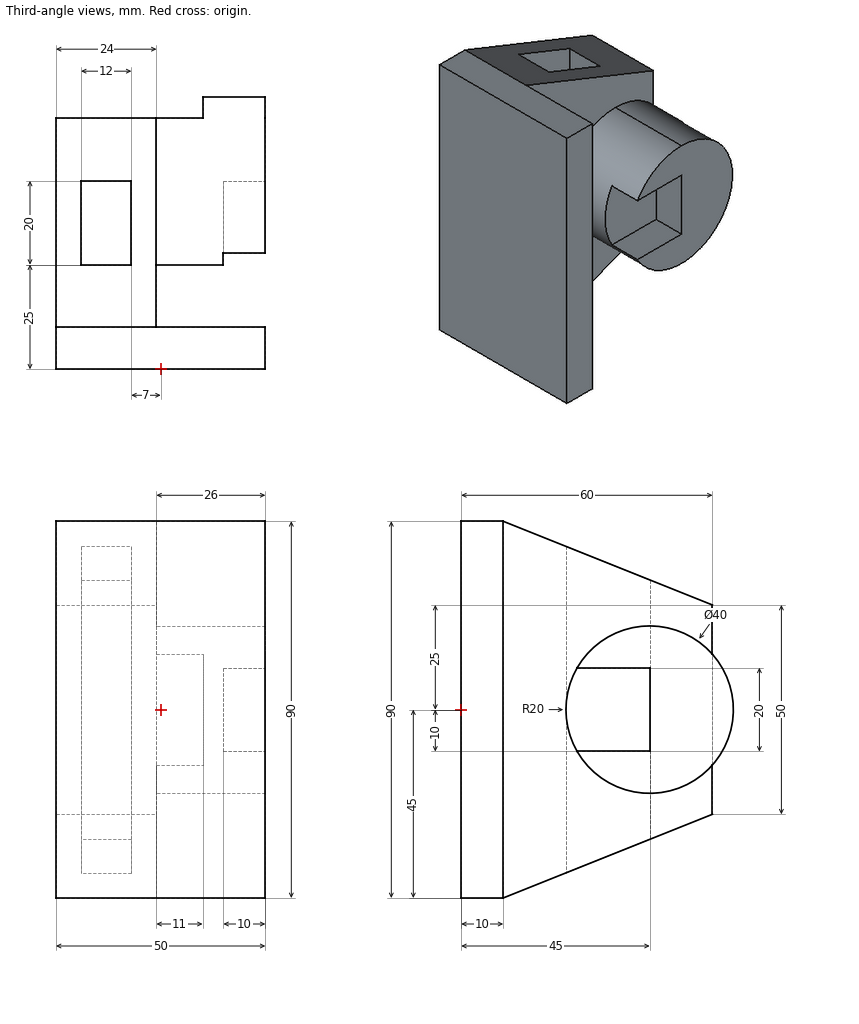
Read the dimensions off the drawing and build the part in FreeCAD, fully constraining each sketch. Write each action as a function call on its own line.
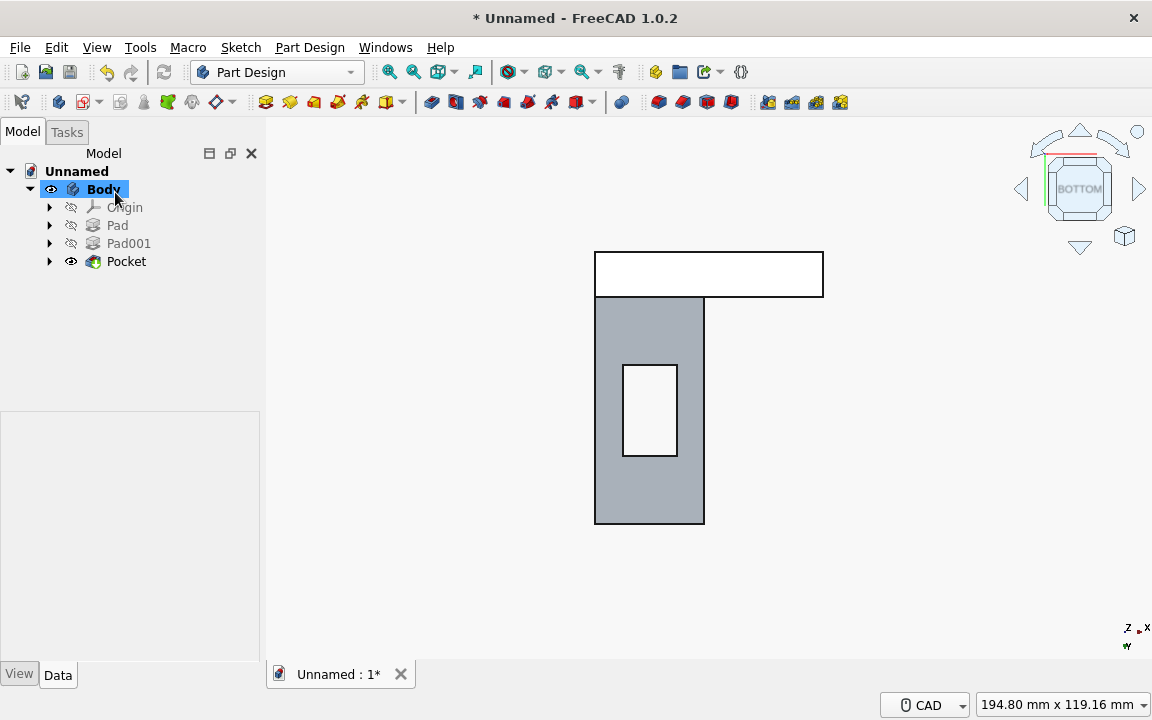
key(0)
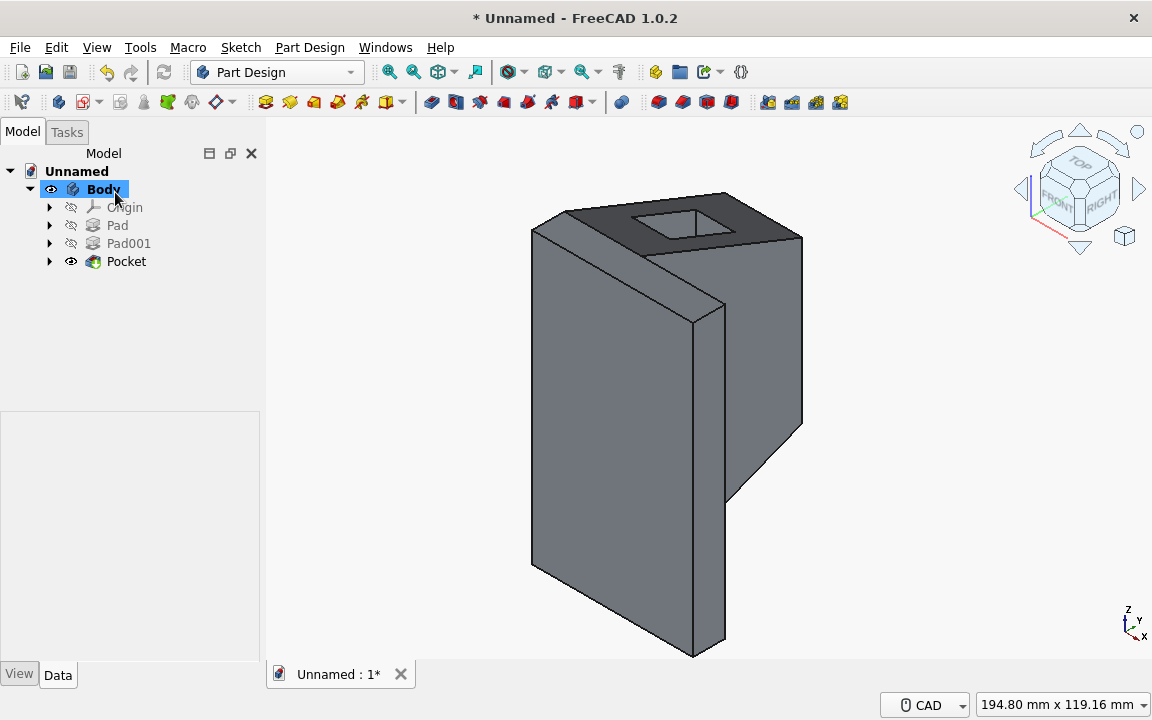
click(745, 410)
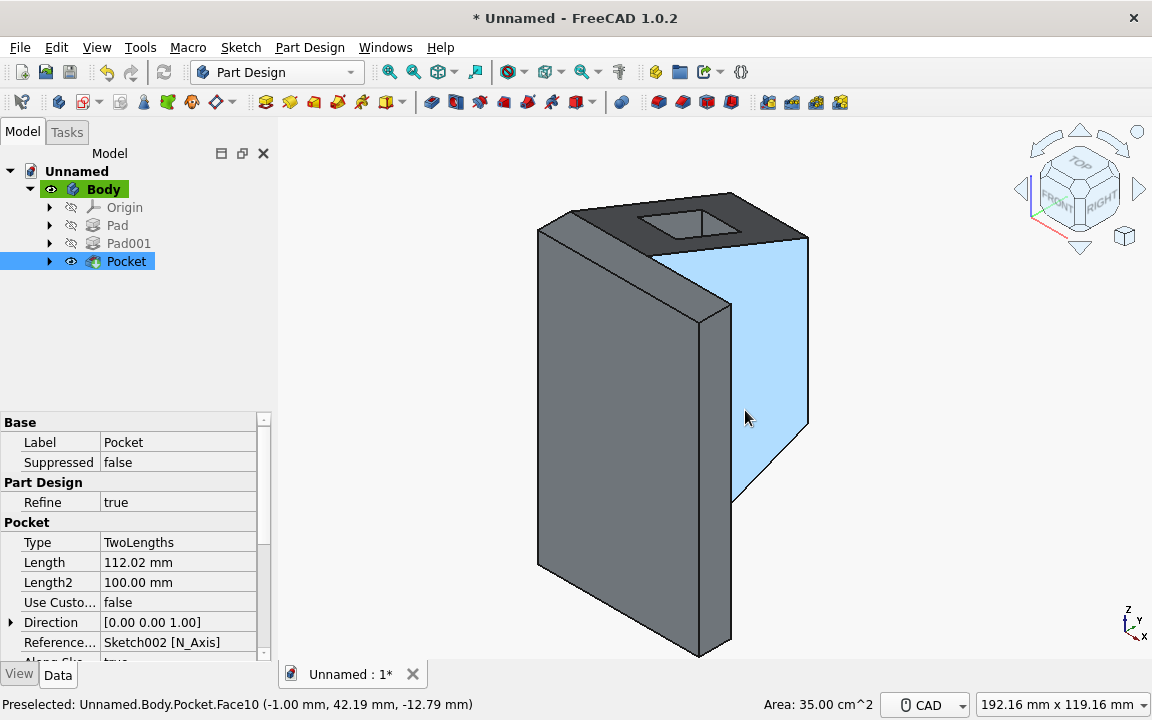
click(84, 102)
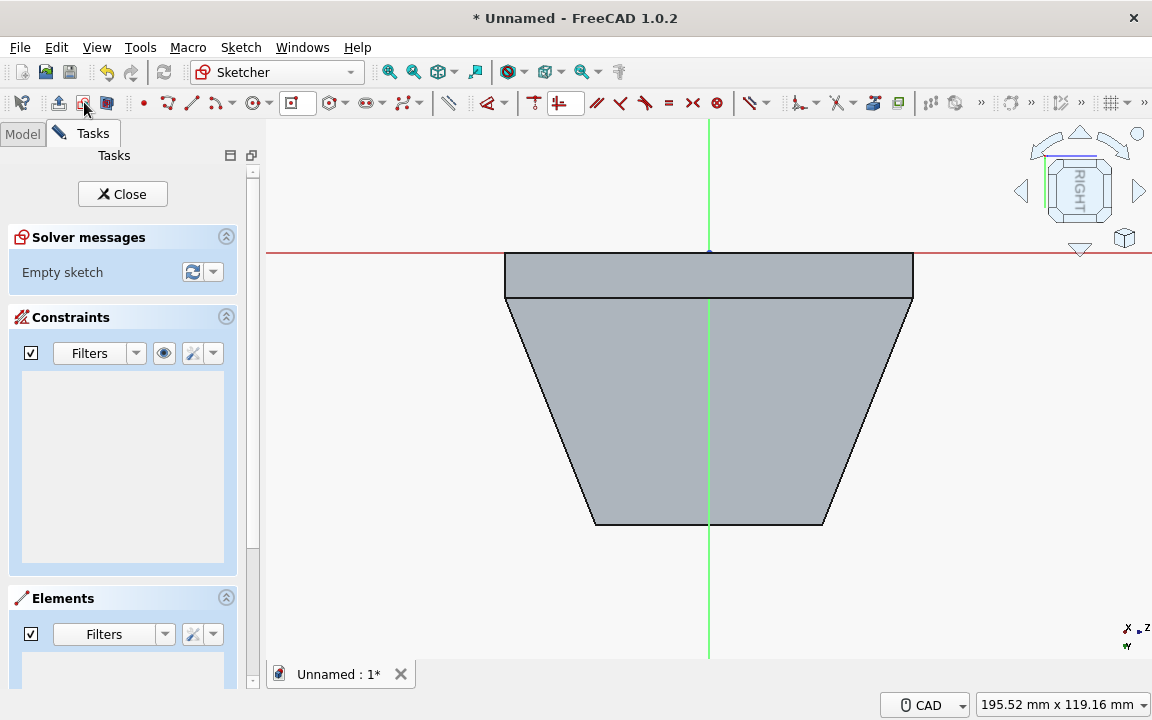
click(108, 104)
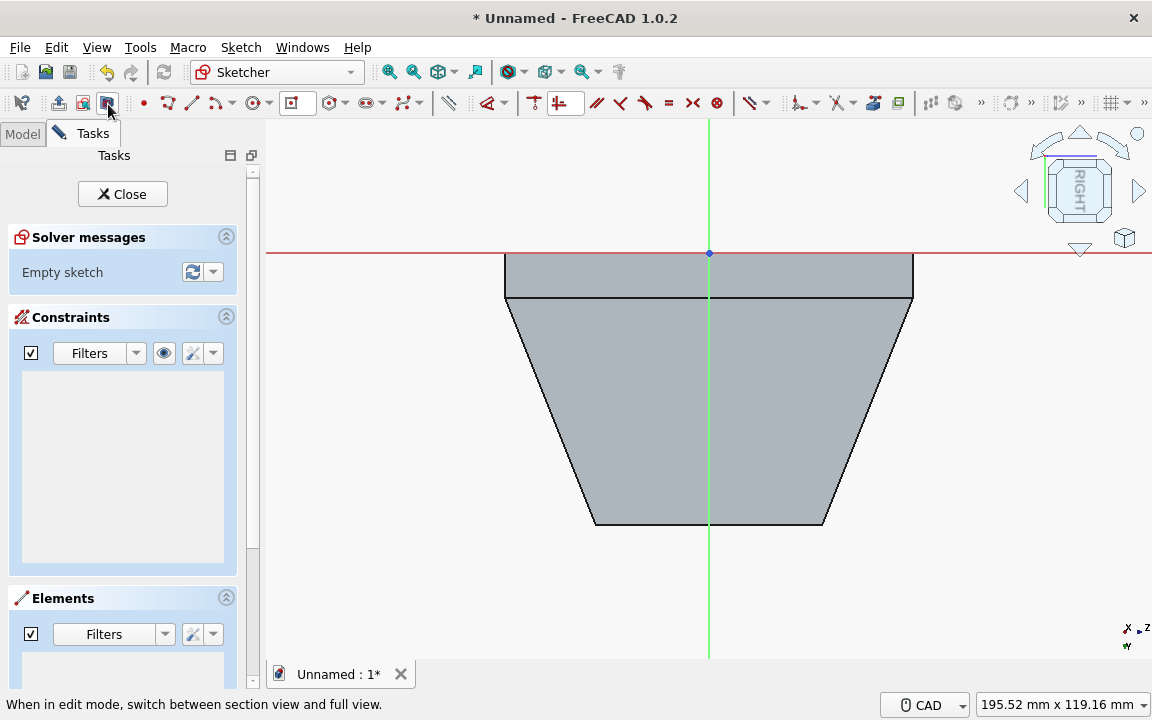
click(254, 104)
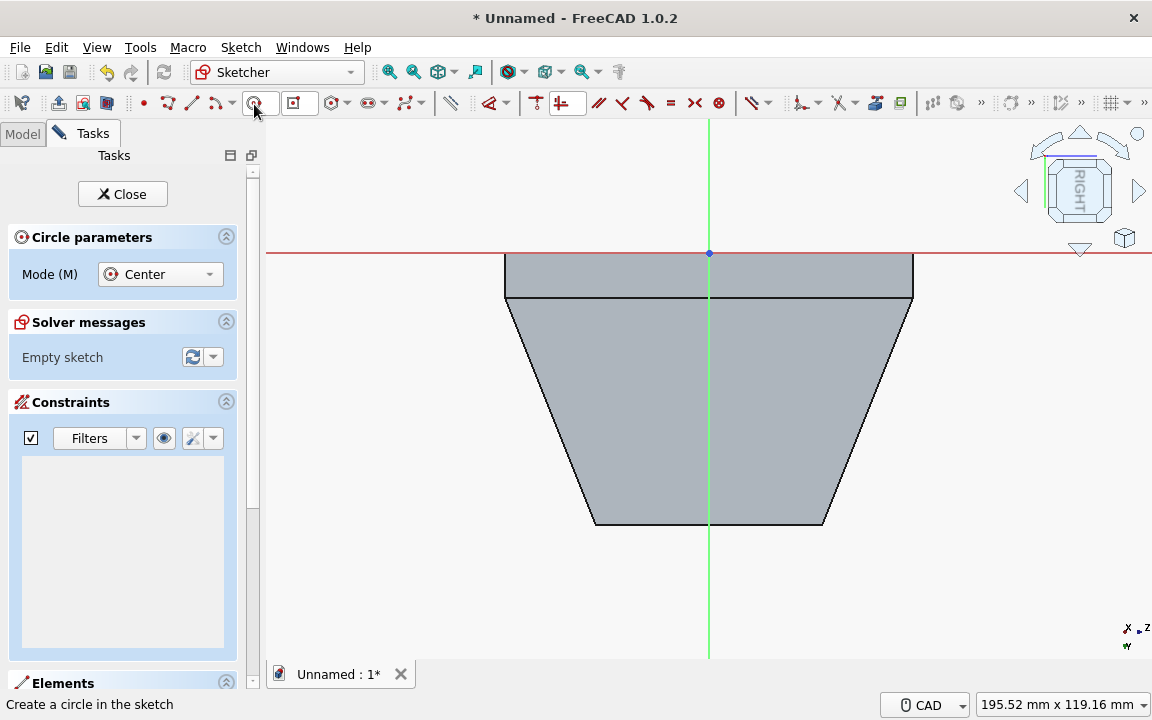
click(709, 457)
move(773, 393)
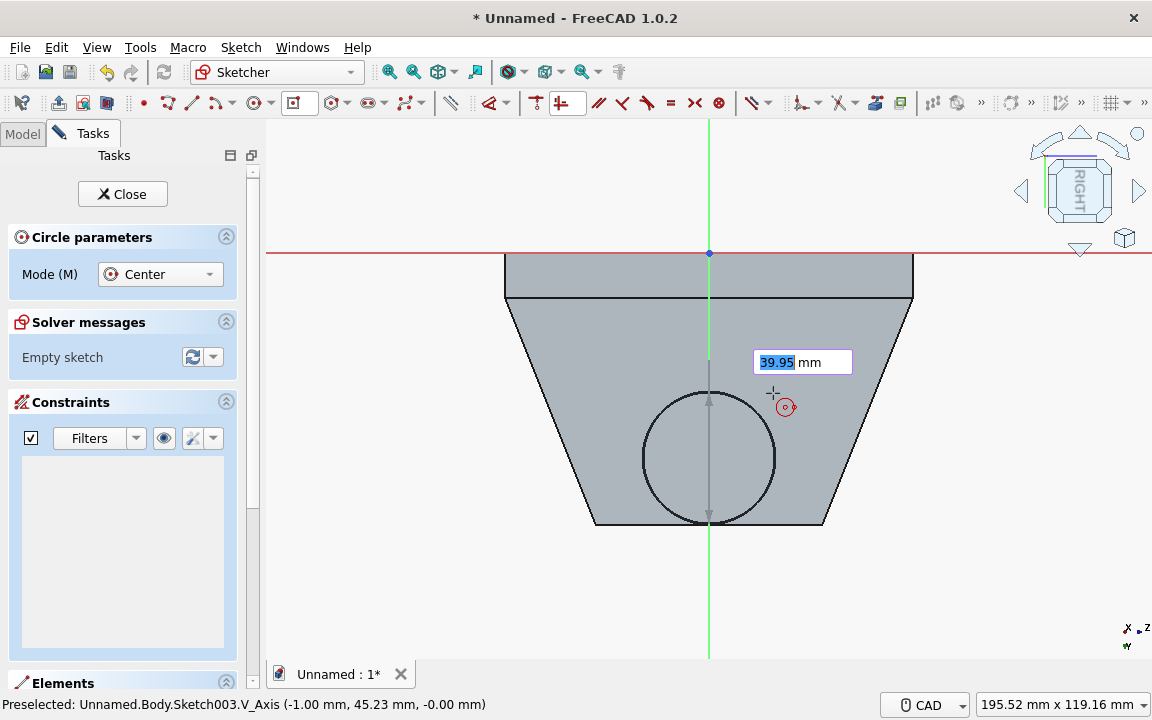
text(40)
key(Return)
key(Escape)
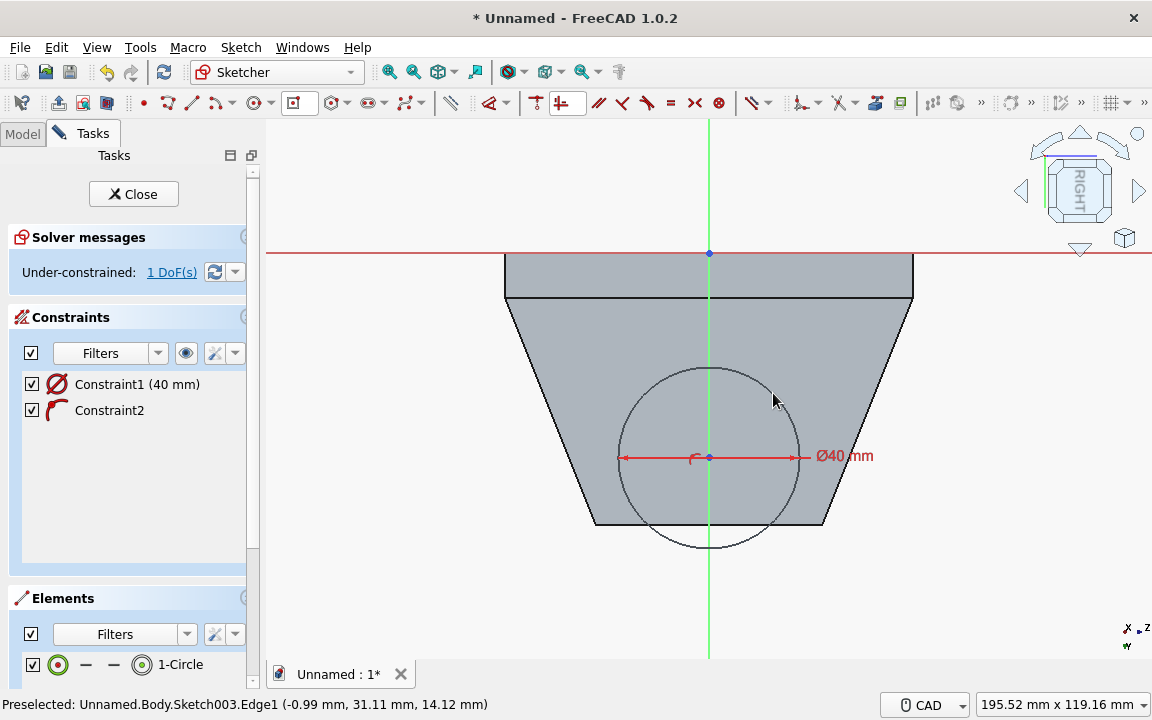
click(490, 104)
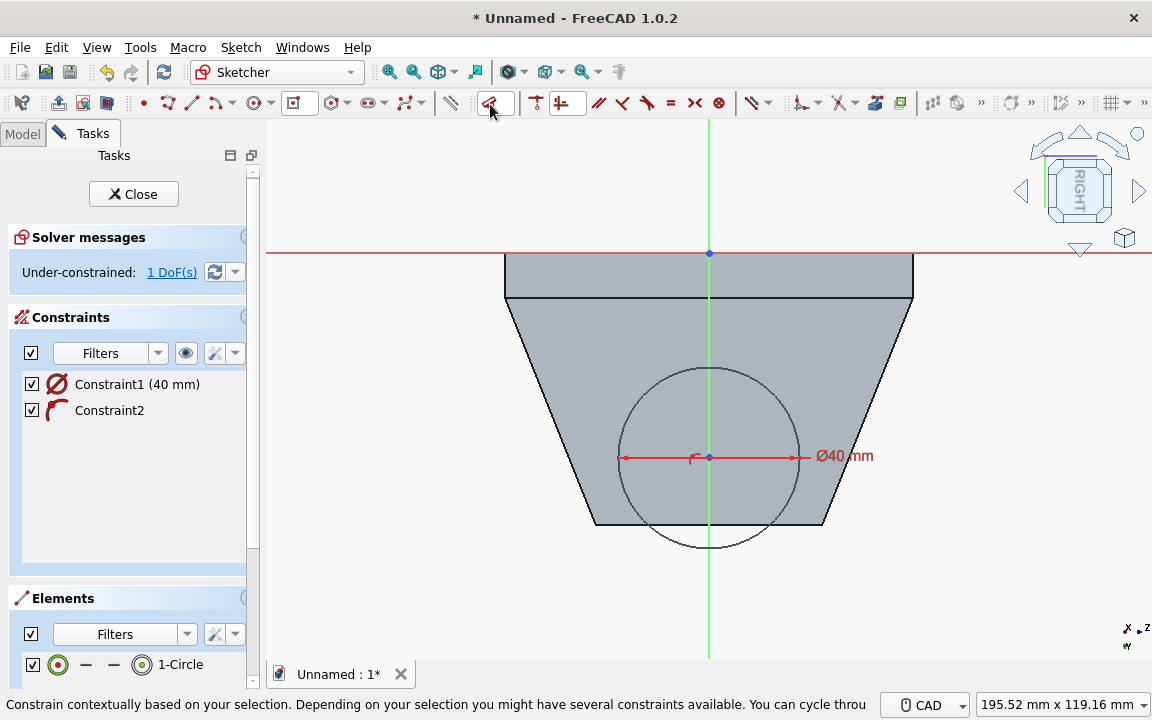
click(709, 458)
click(743, 356)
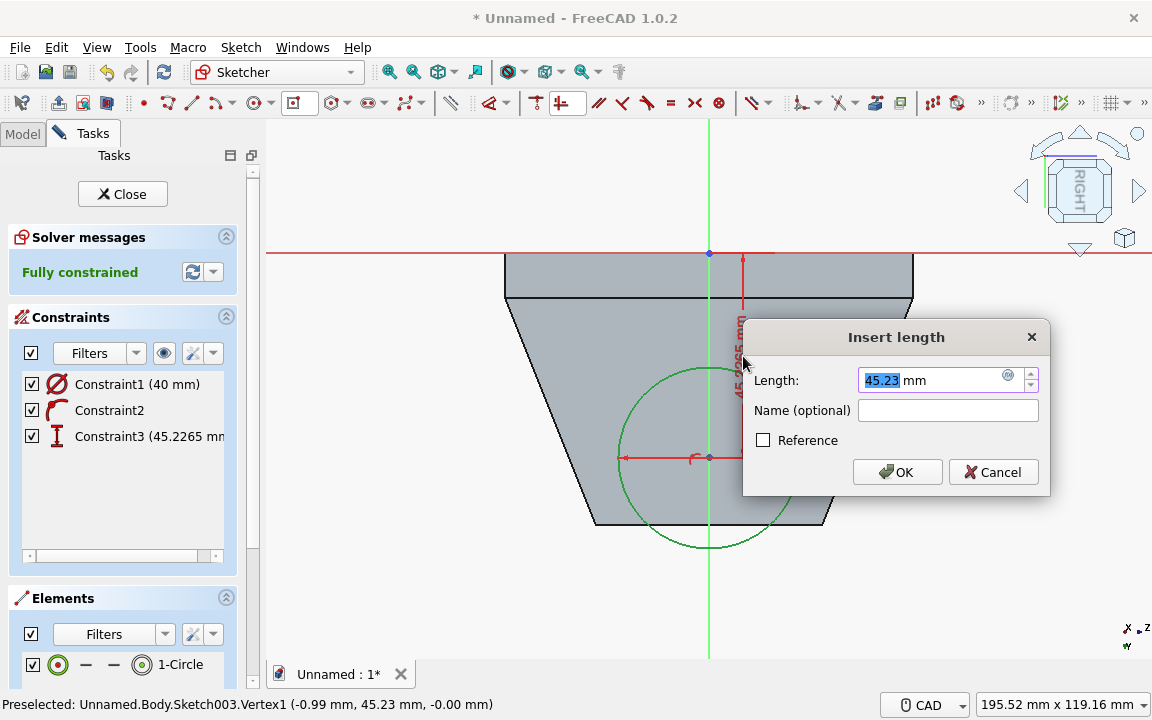
text(45)
key(Return)
key(Escape)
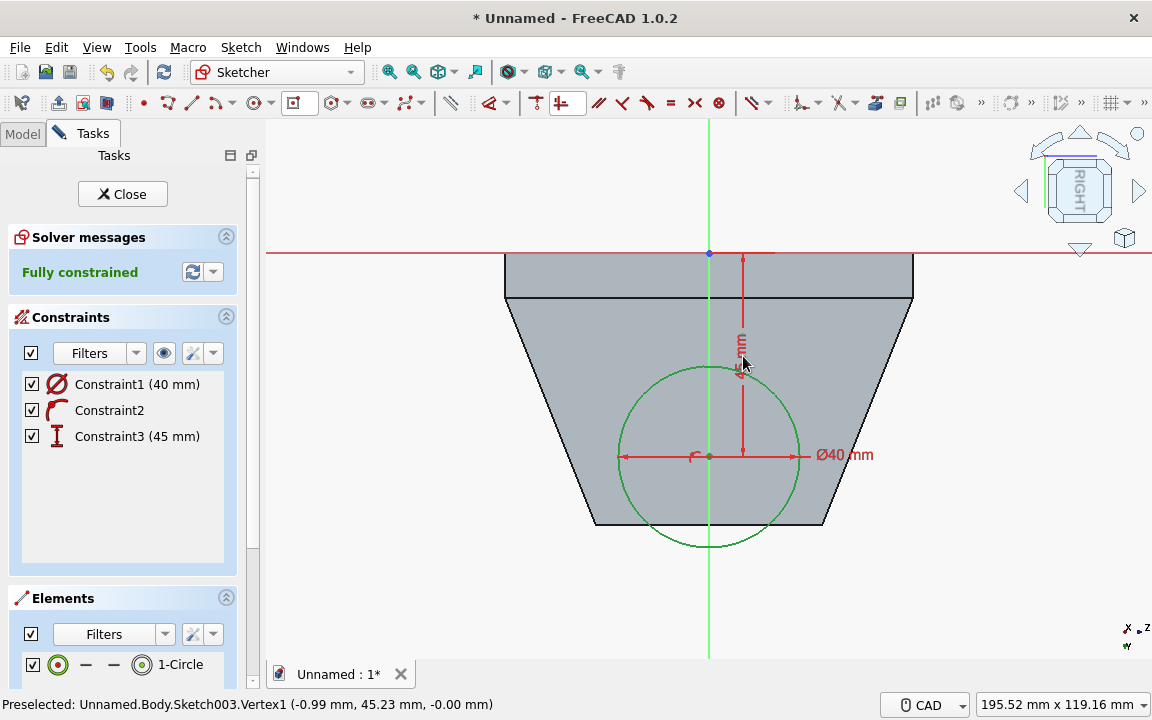
click(123, 194)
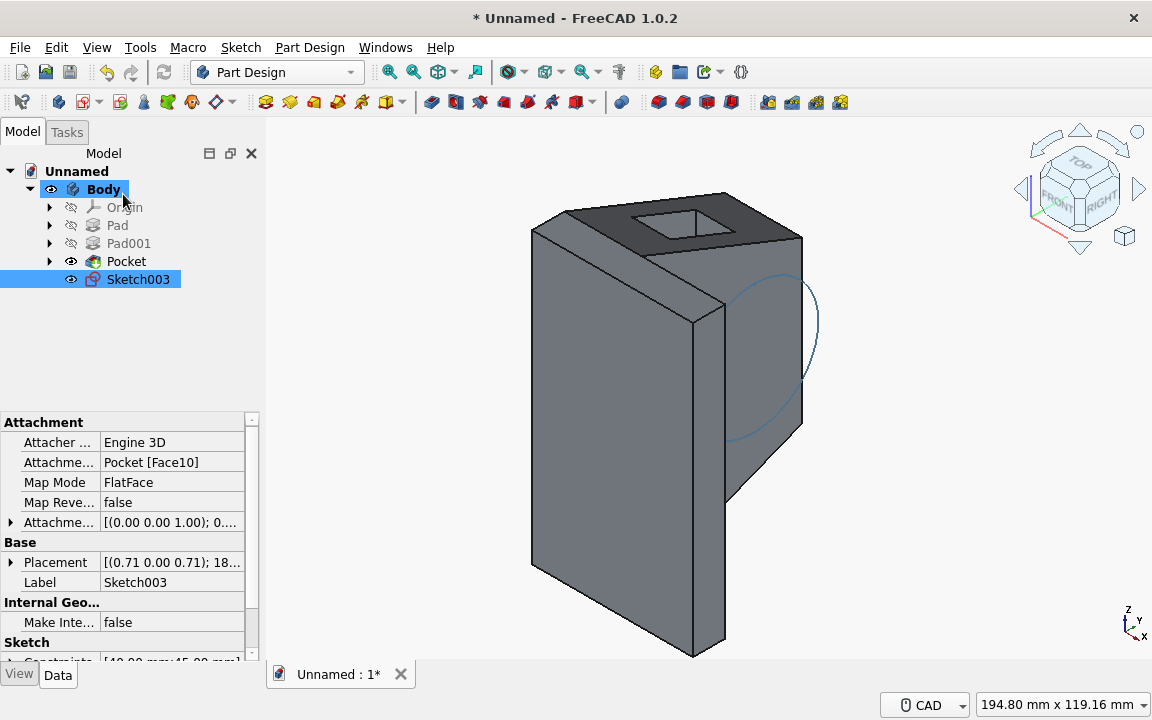
click(266, 102)